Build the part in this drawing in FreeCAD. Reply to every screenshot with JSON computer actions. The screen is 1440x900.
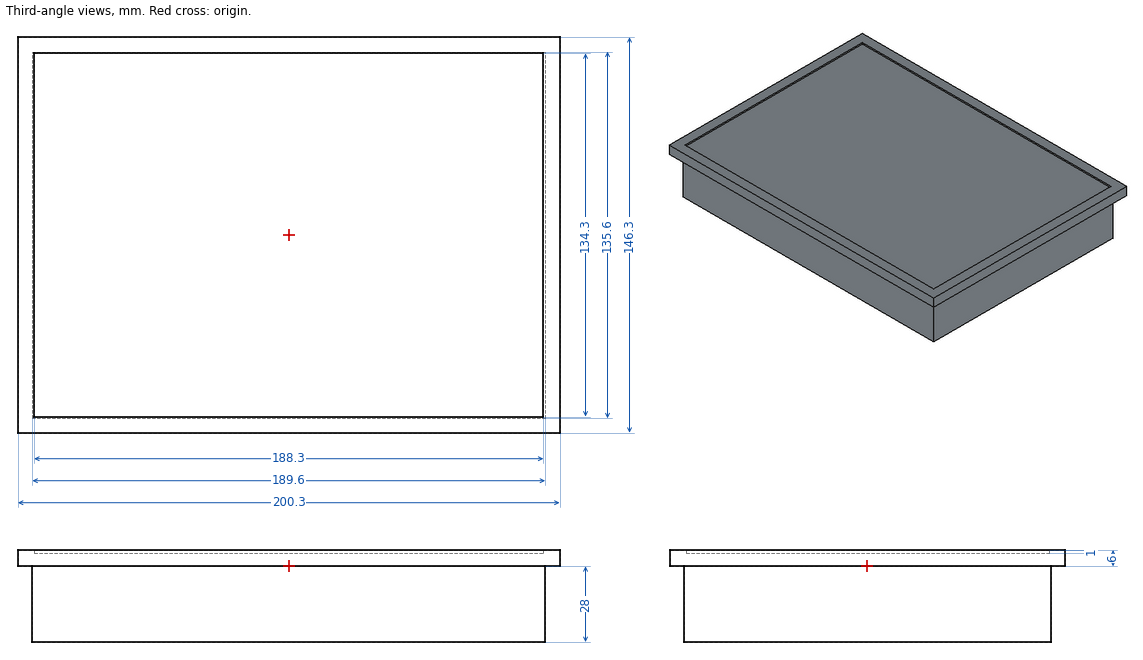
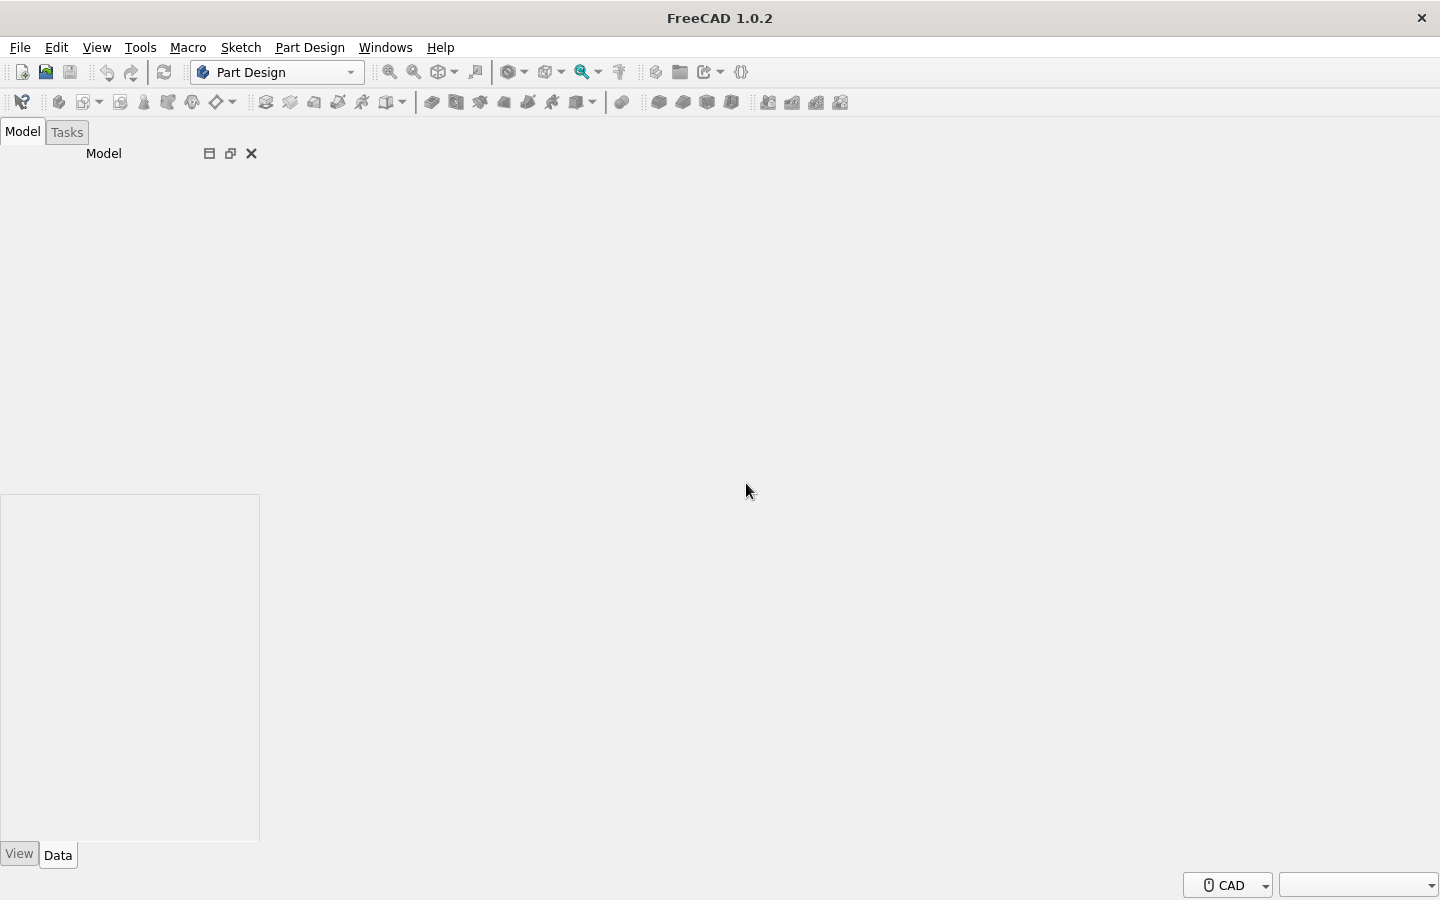
{"action": "left_click", "coordinate": [22, 72]}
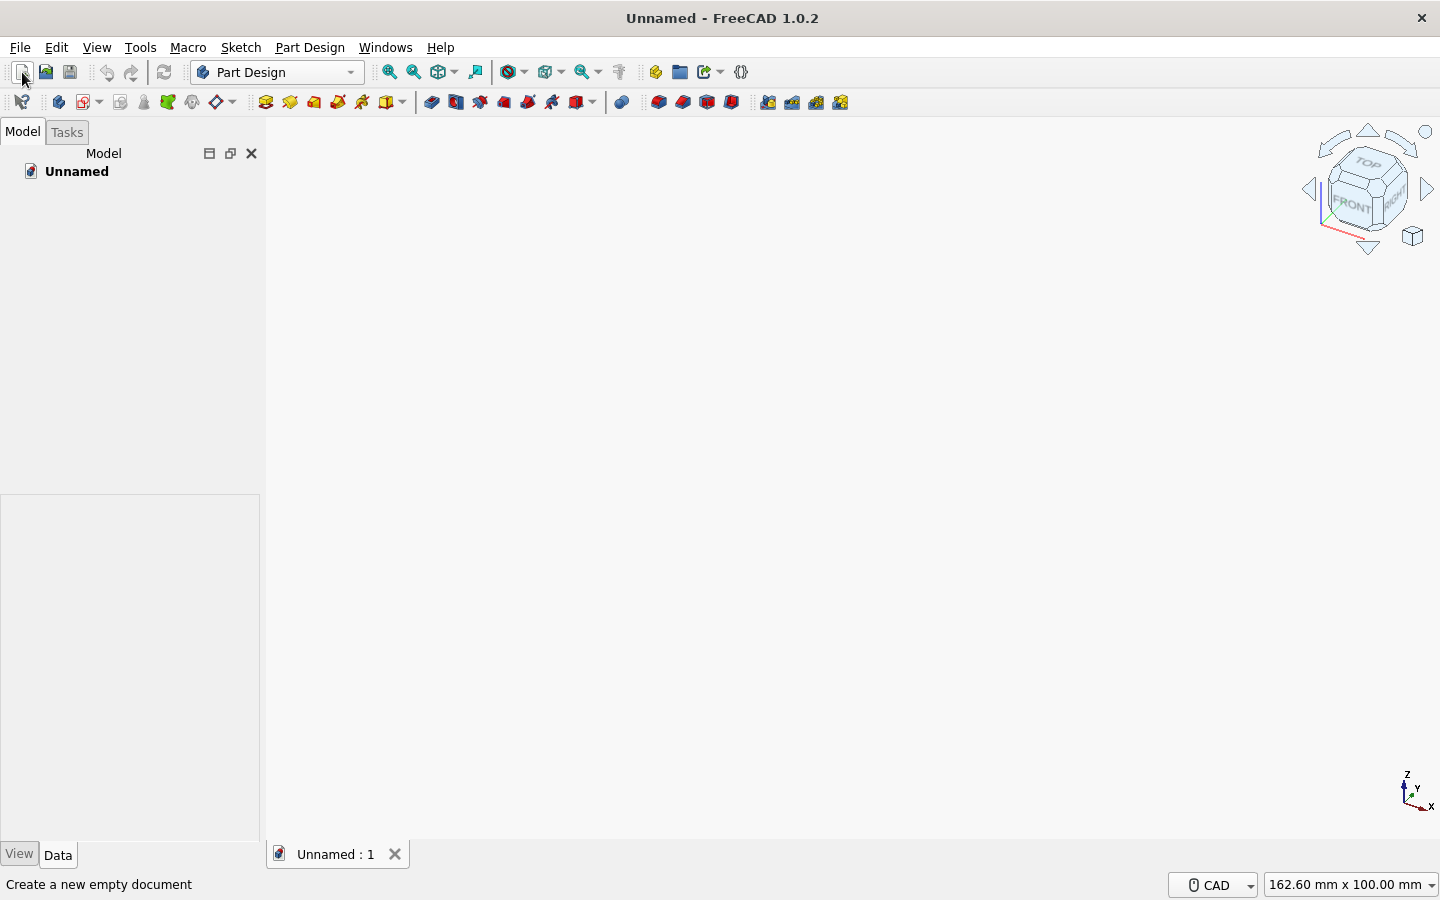
{"action": "left_click", "coordinate": [84, 102]}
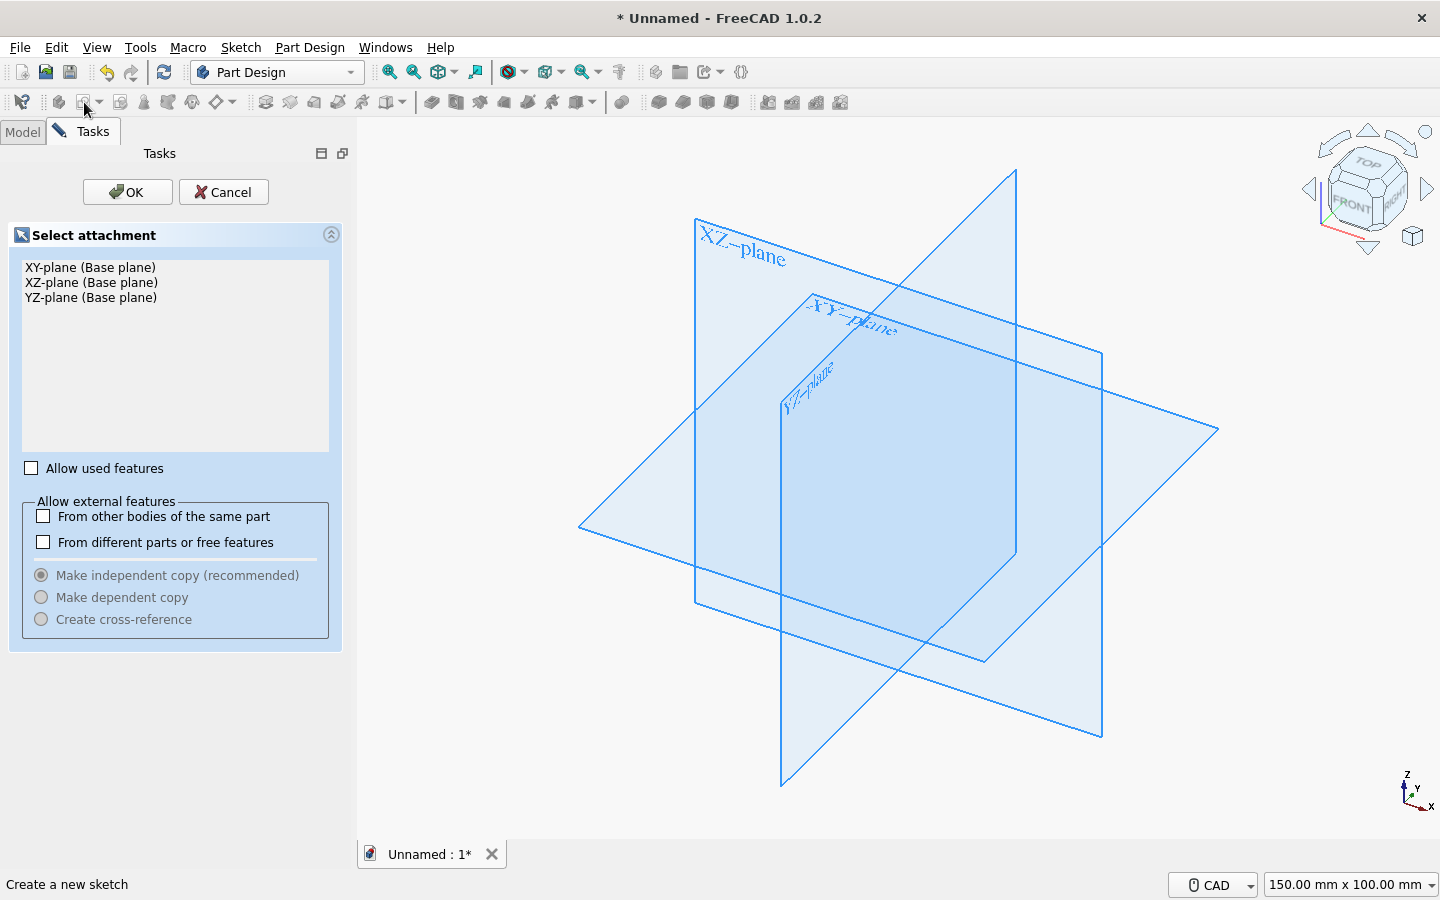
{"action": "left_click", "coordinate": [82, 268]}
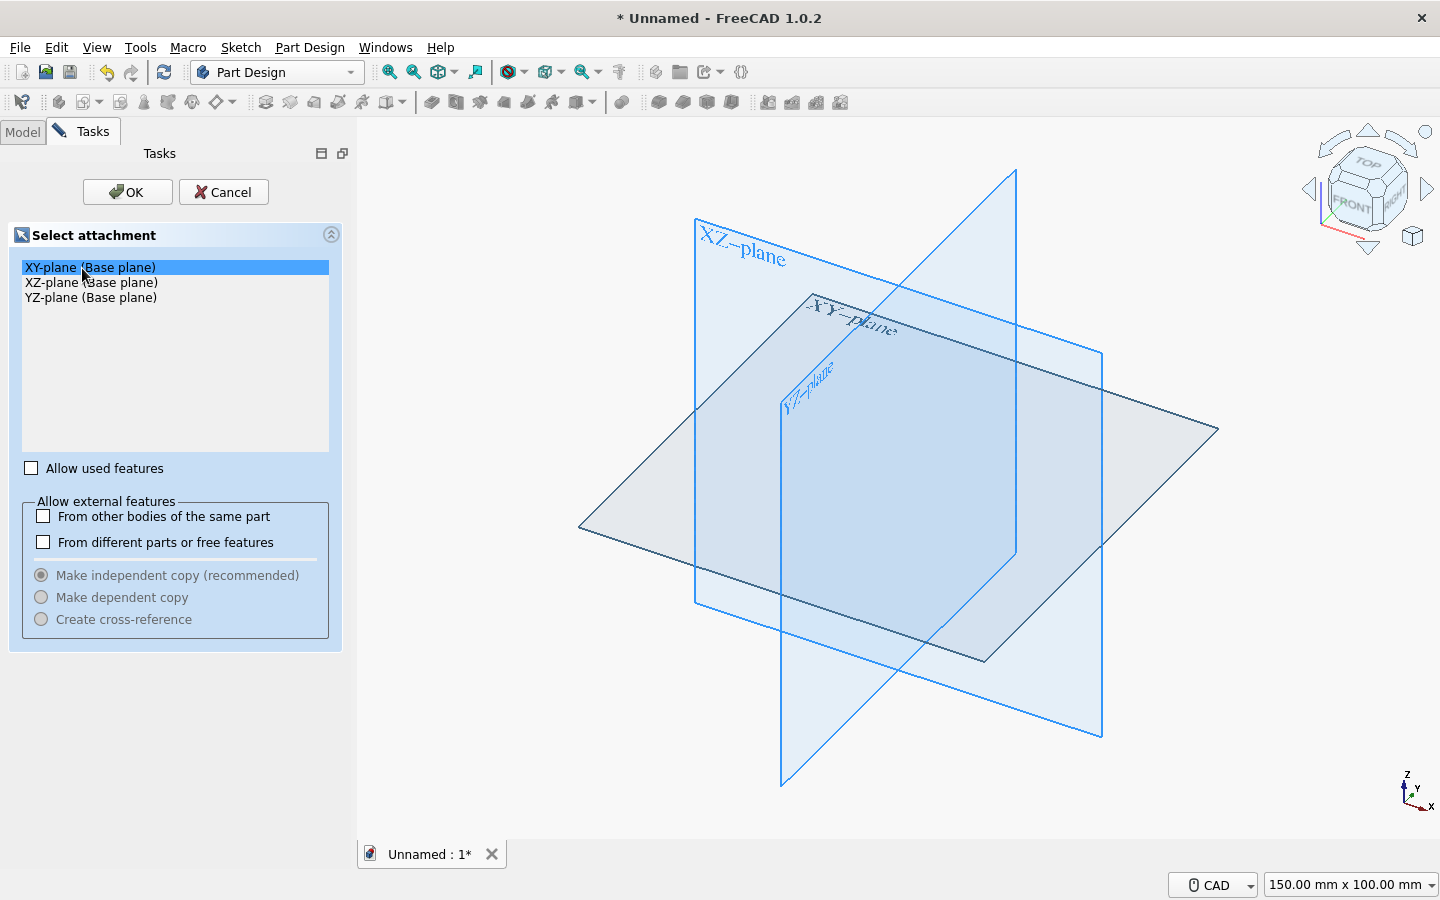
{"action": "left_click", "coordinate": [128, 192]}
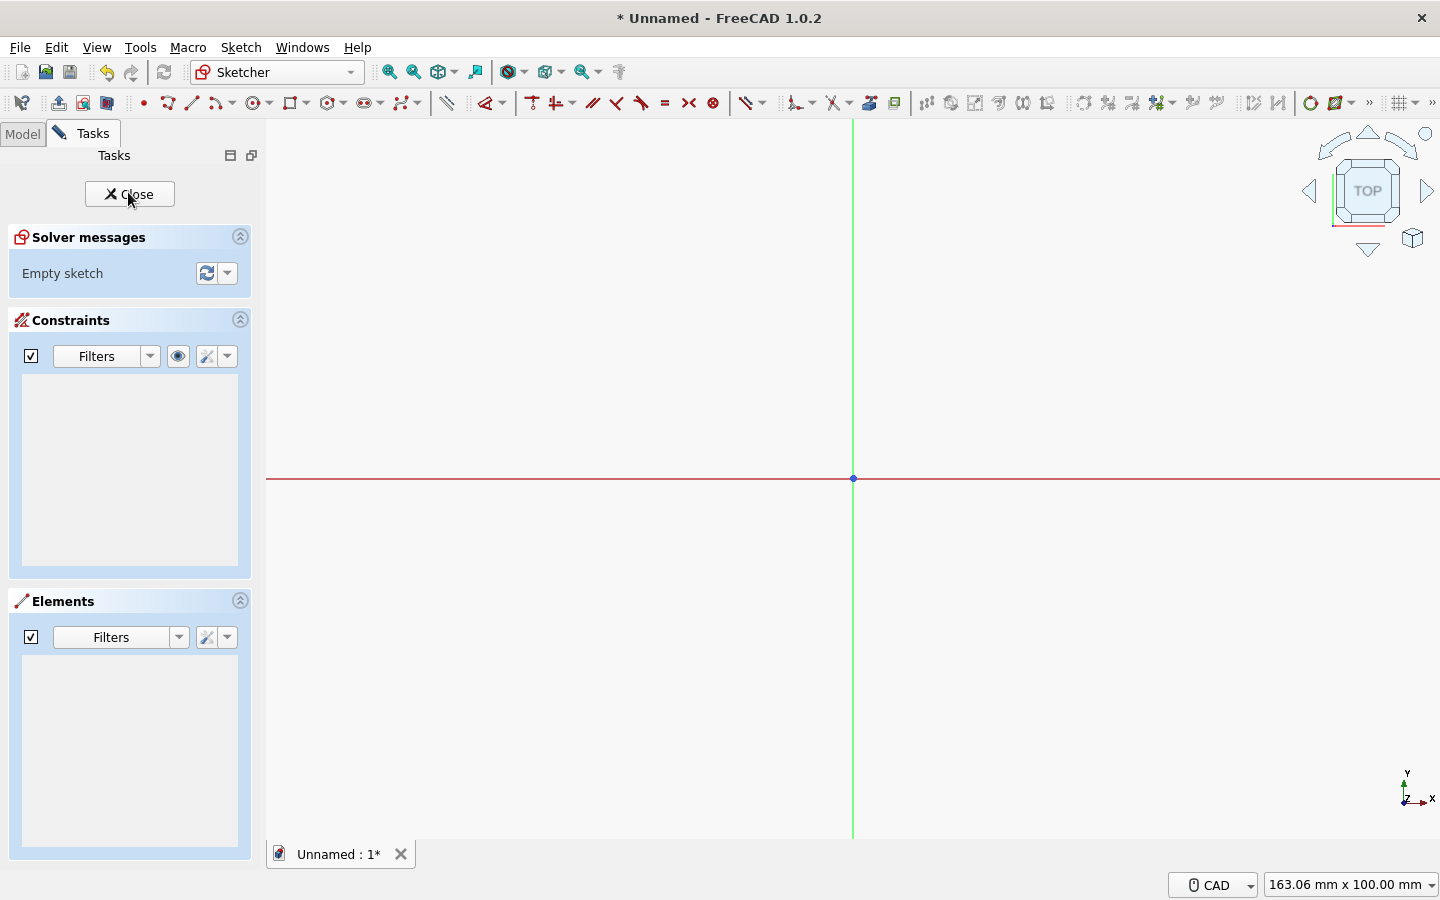
{"action": "scroll", "coordinate": [729, 479], "scroll_direction": "down", "scroll_amount": 4}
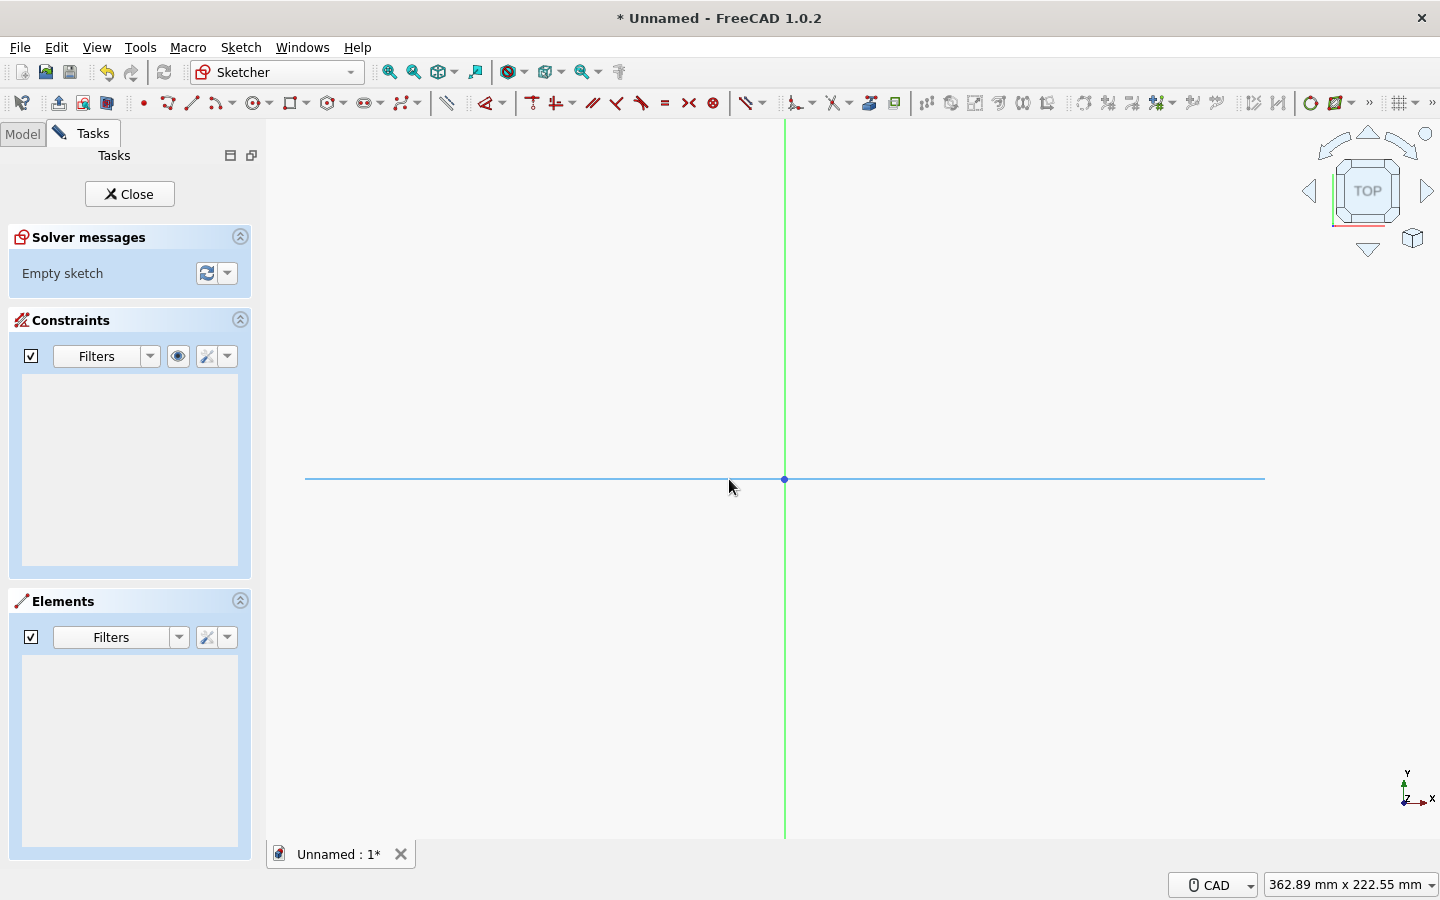
{"action": "key", "text": "g v"}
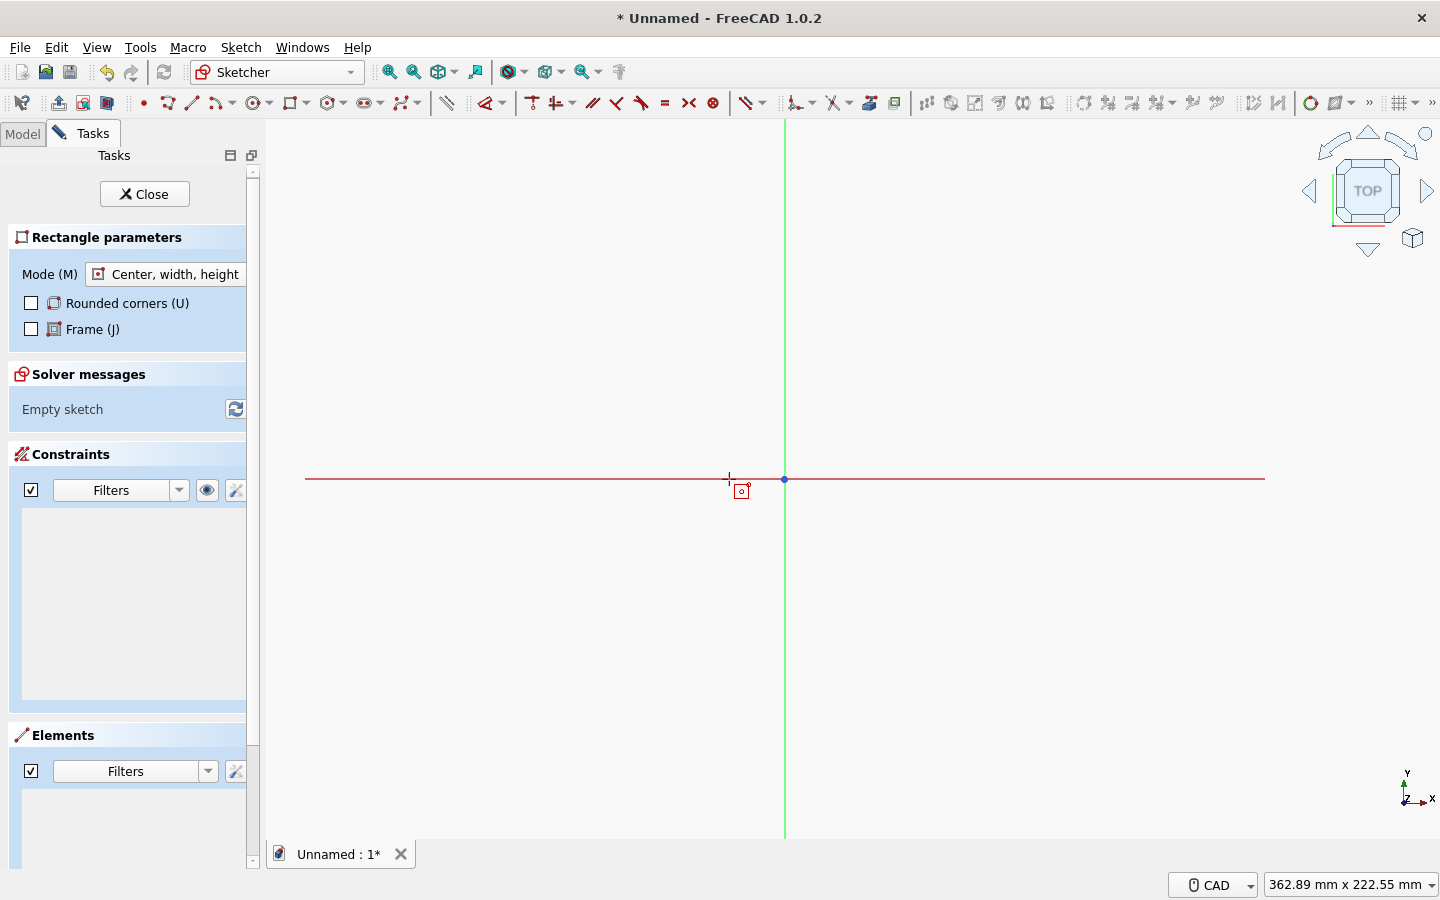
{"action": "left_click", "coordinate": [785, 479]}
{"action": "left_click", "coordinate": [1109, 243]}
{"action": "key", "text": "Escape"}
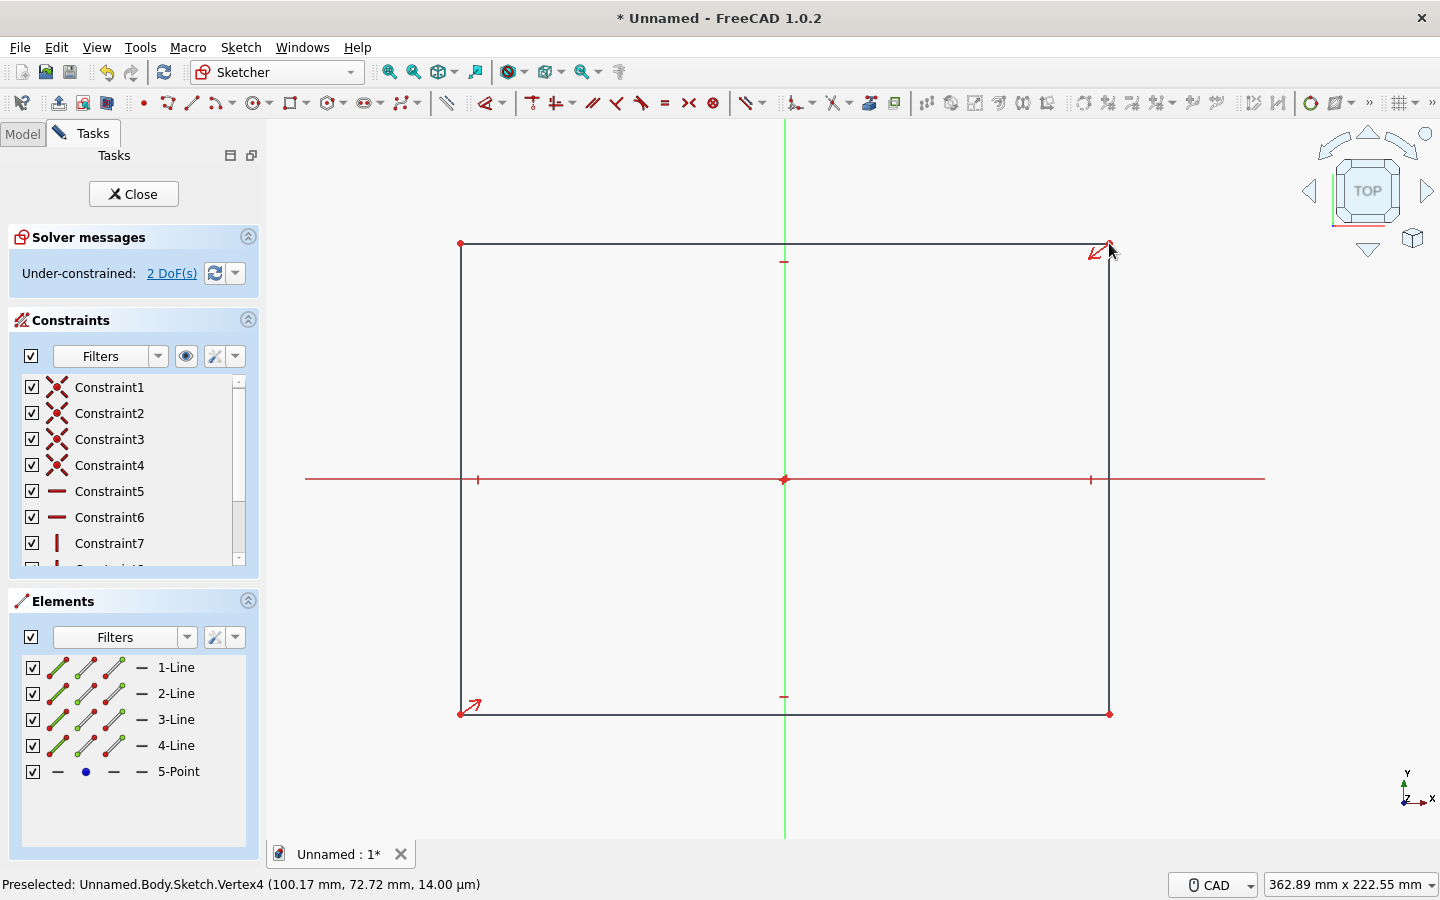
{"action": "left_click", "coordinate": [486, 104]}